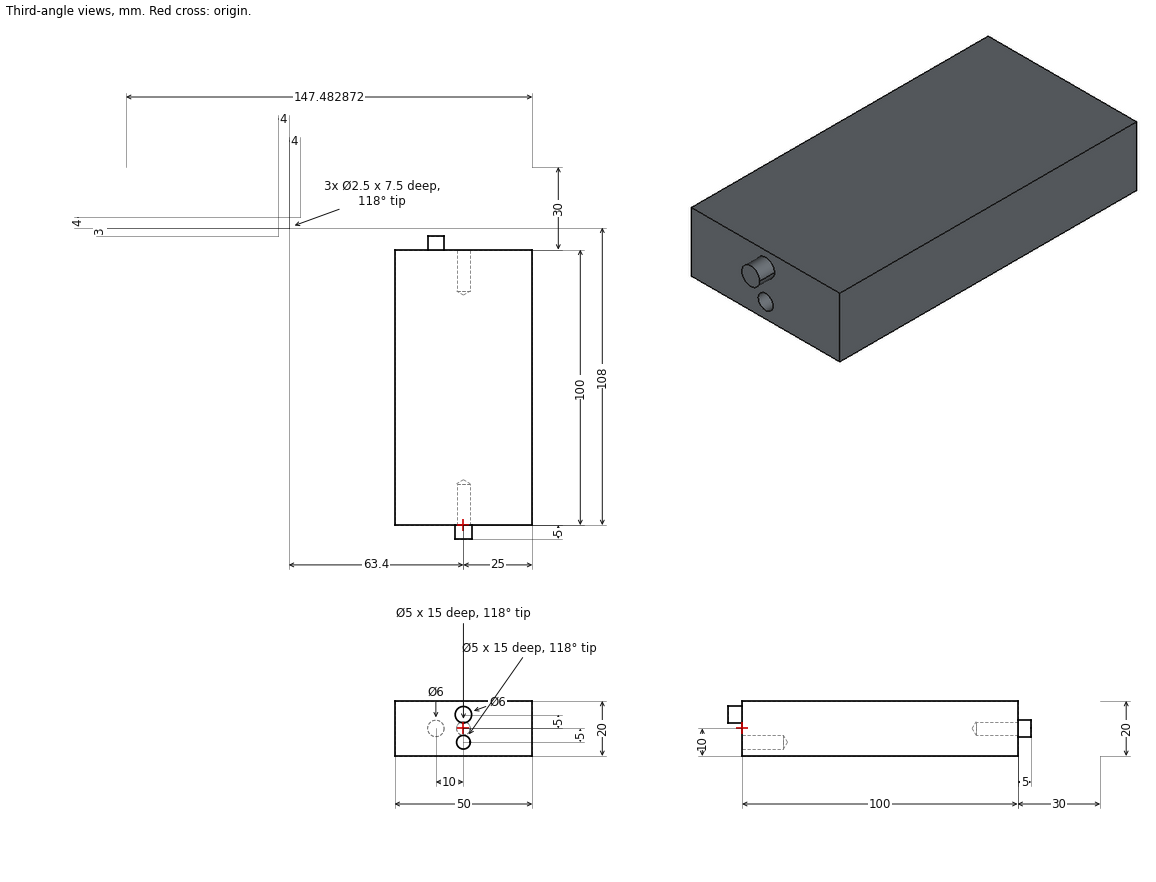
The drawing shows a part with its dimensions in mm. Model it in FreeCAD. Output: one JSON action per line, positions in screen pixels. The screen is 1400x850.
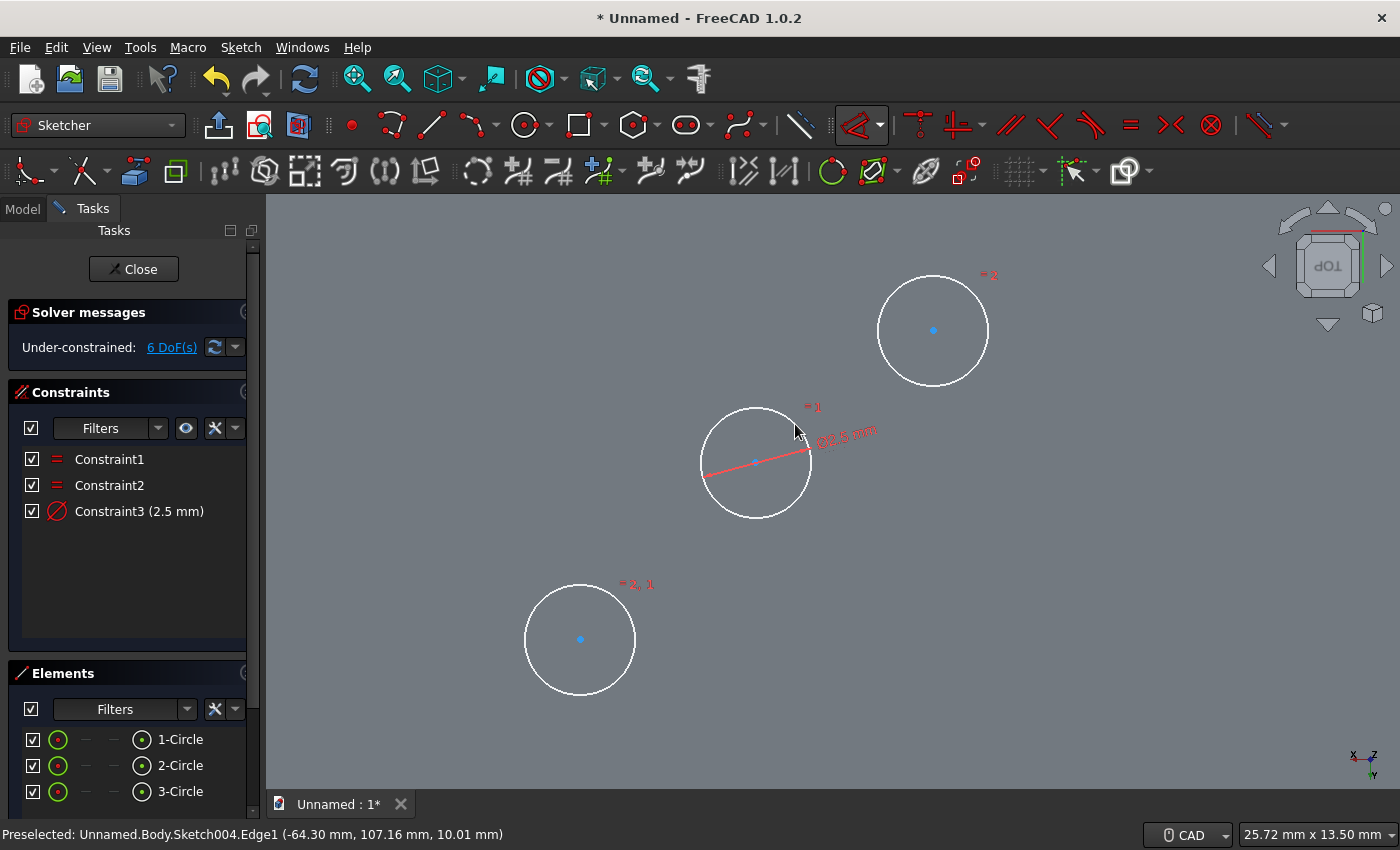
{"action": "left_click", "coordinate": [756, 463]}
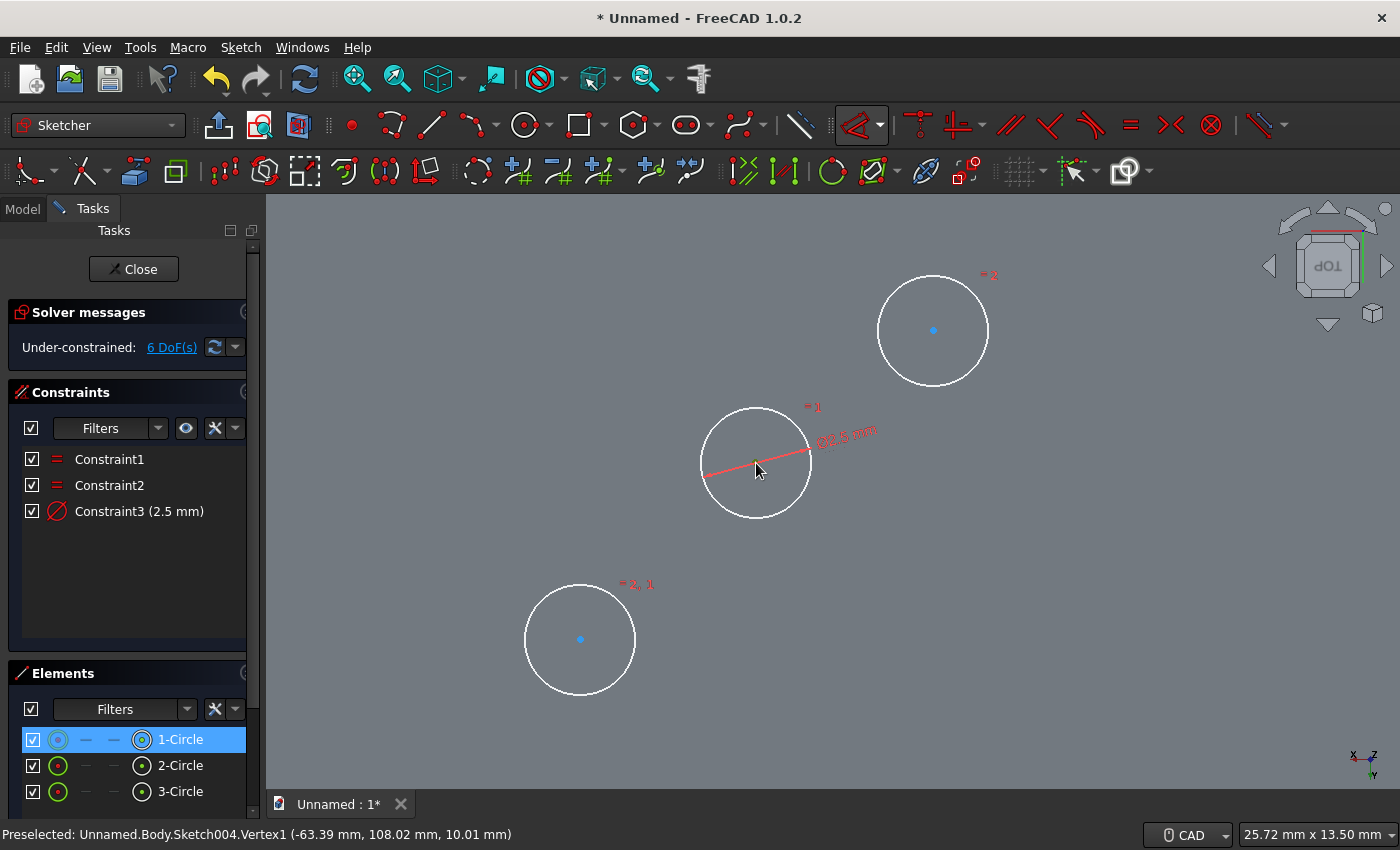
{"action": "left_click", "coordinate": [580, 640]}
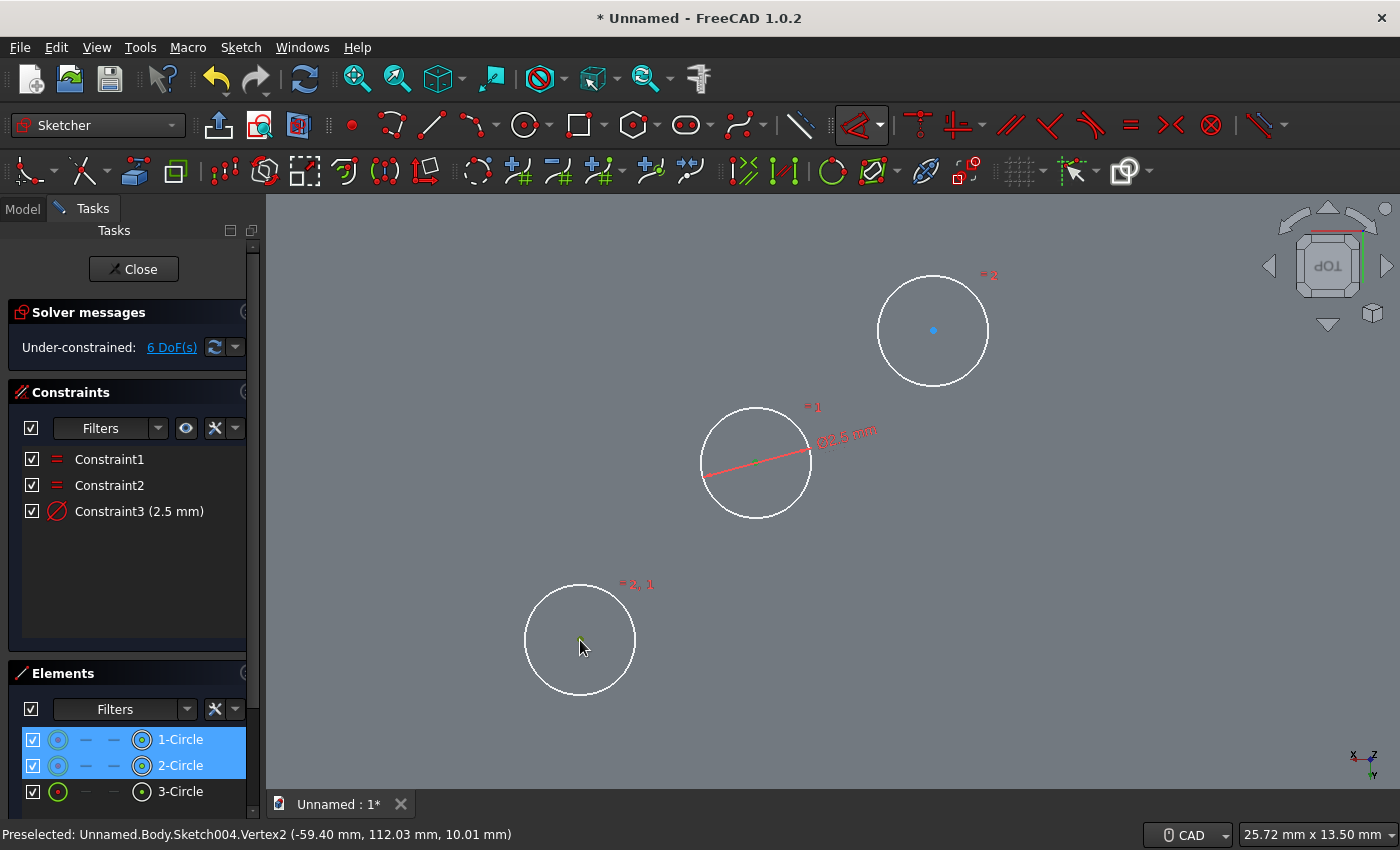
{"action": "left_click", "coordinate": [882, 126]}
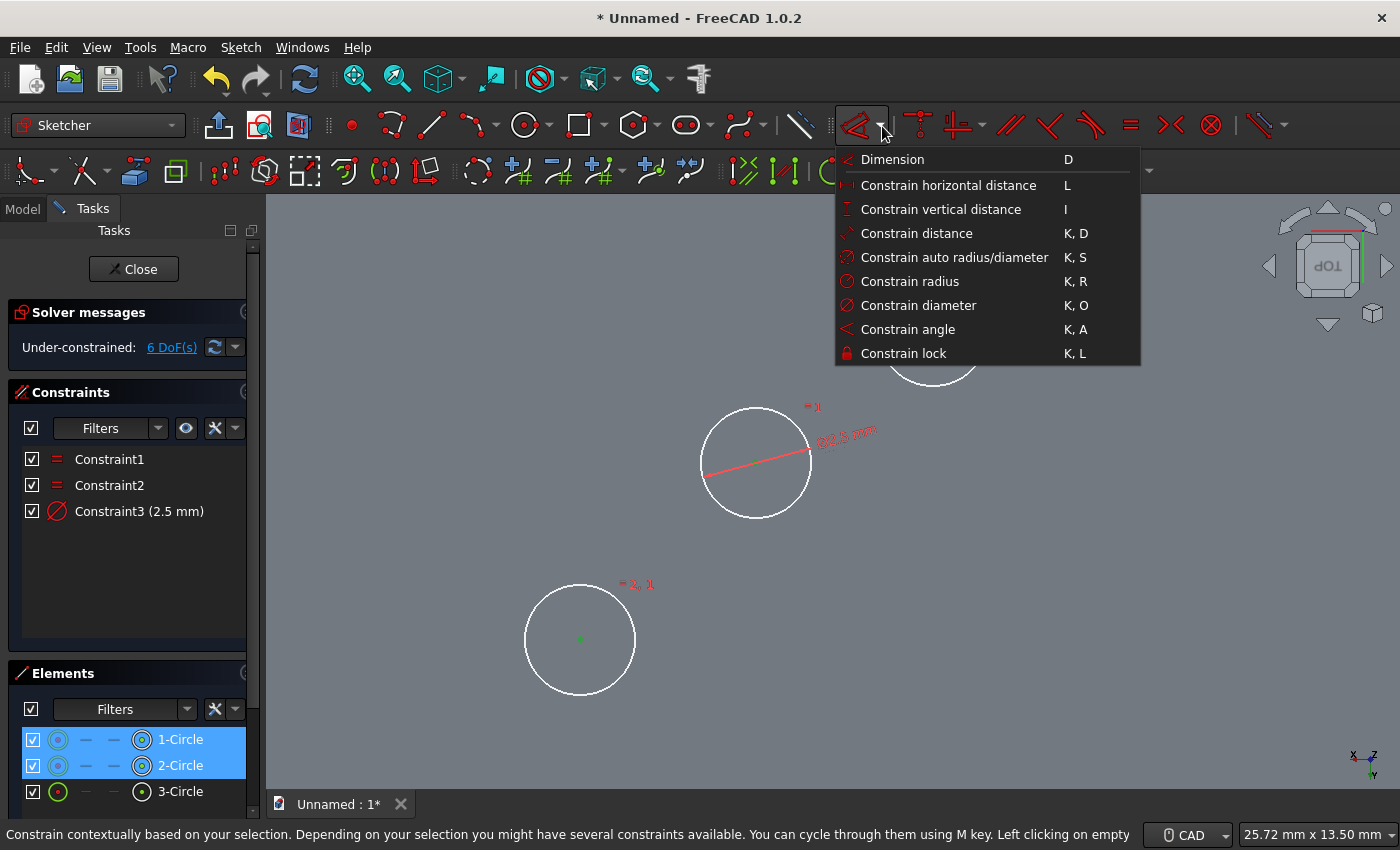
{"action": "left_click", "coordinate": [988, 185]}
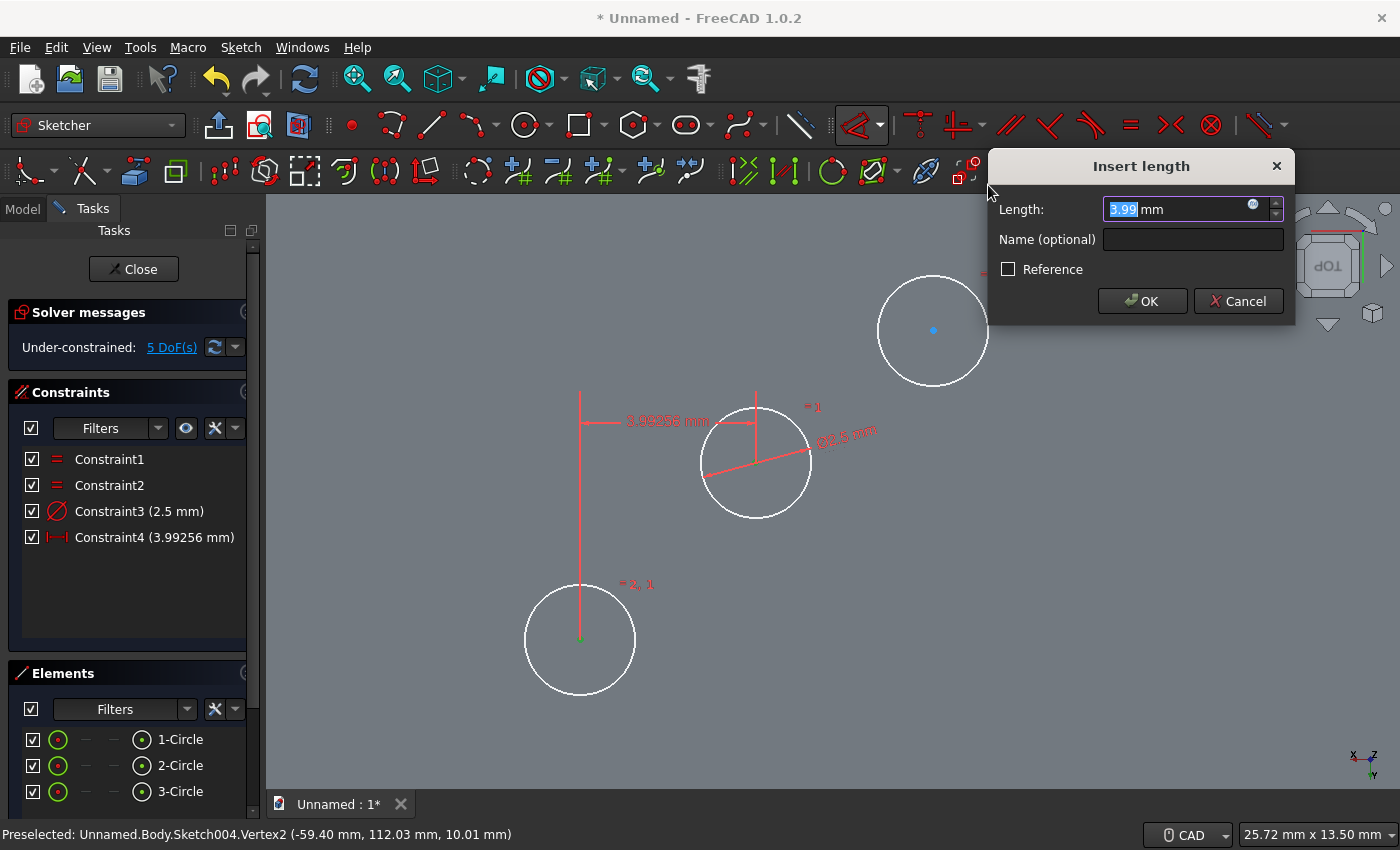
{"action": "type", "text": "4"}
{"action": "key", "text": "Return"}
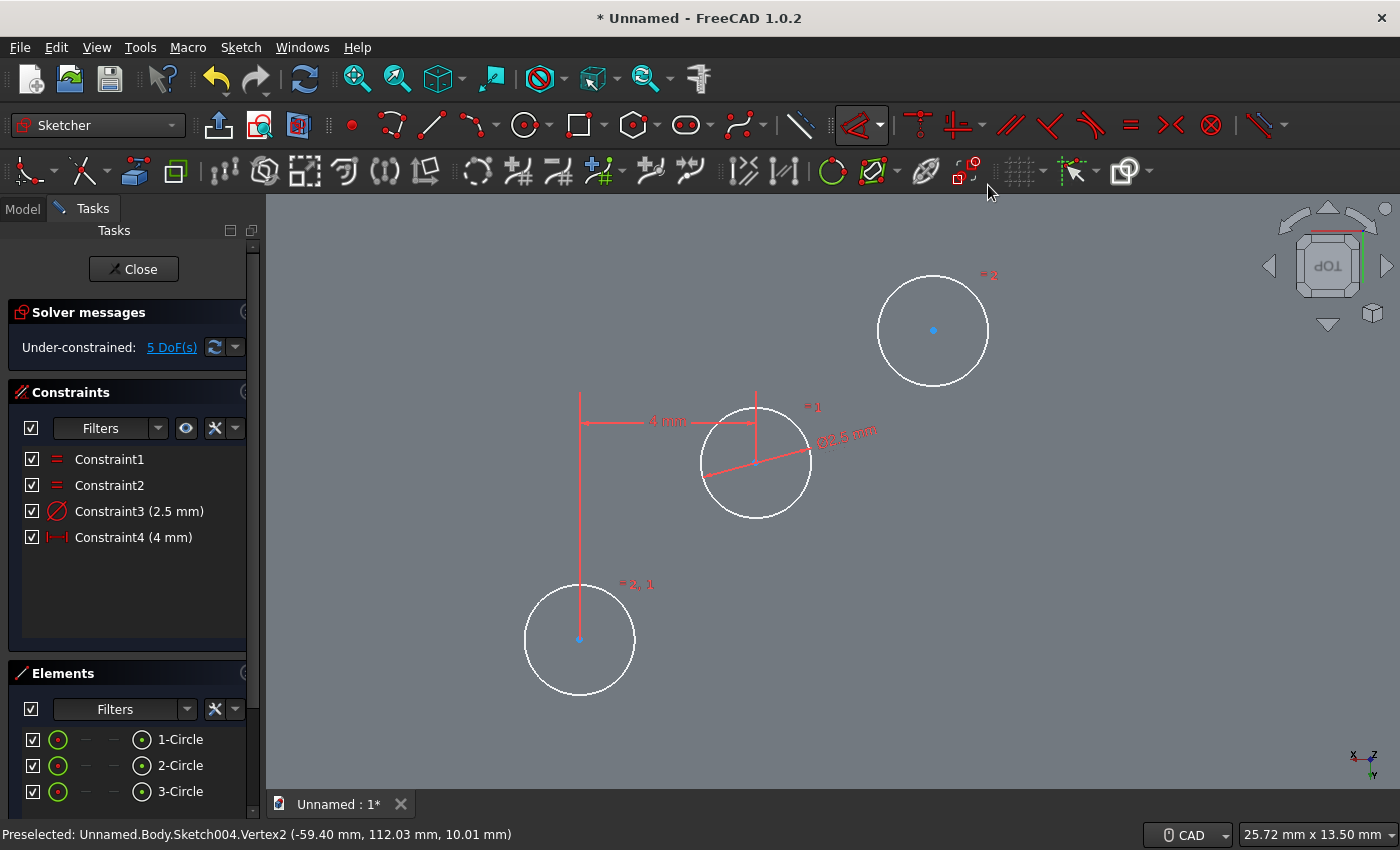
{"action": "left_click", "coordinate": [756, 463]}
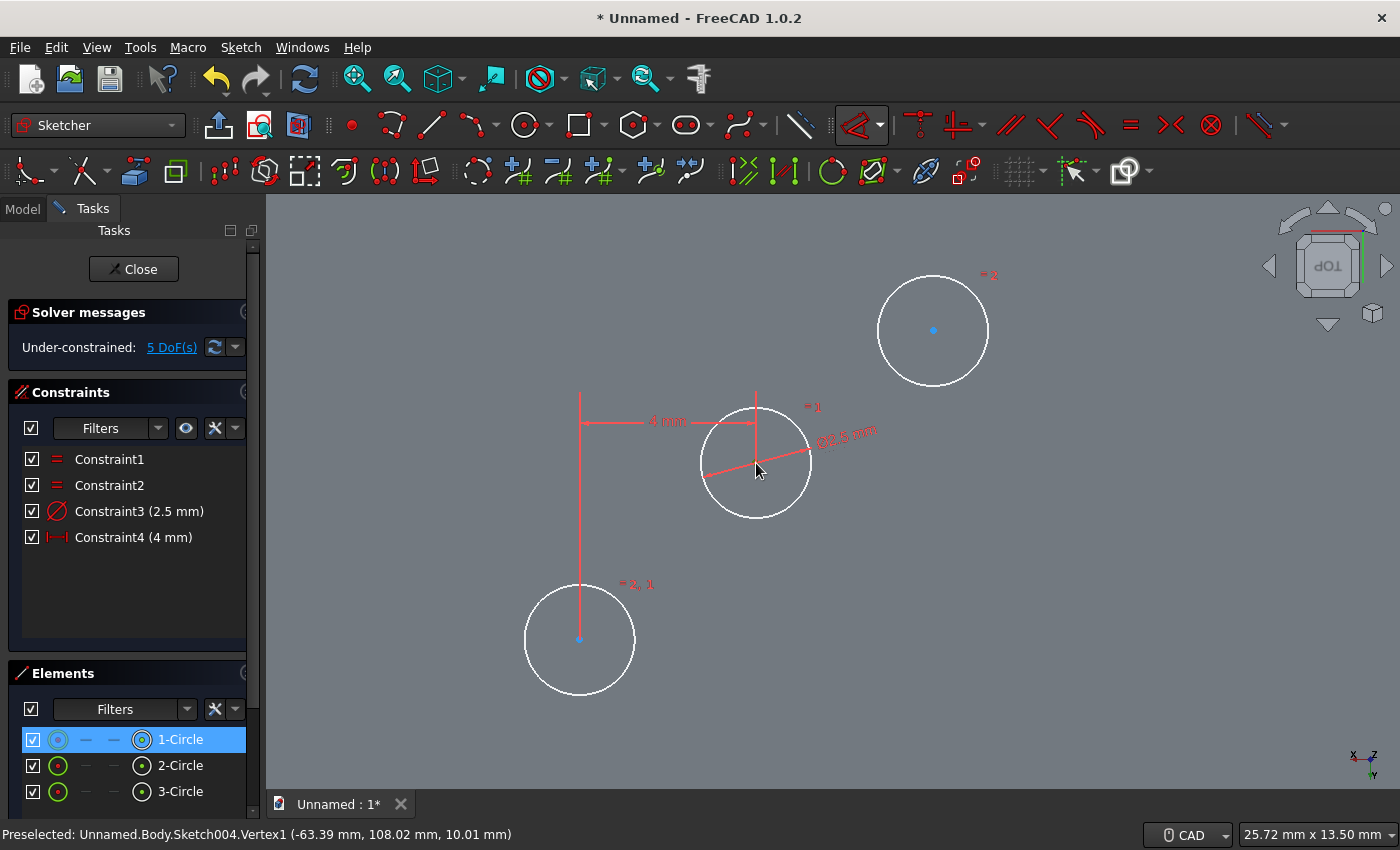
{"action": "left_click", "coordinate": [580, 640]}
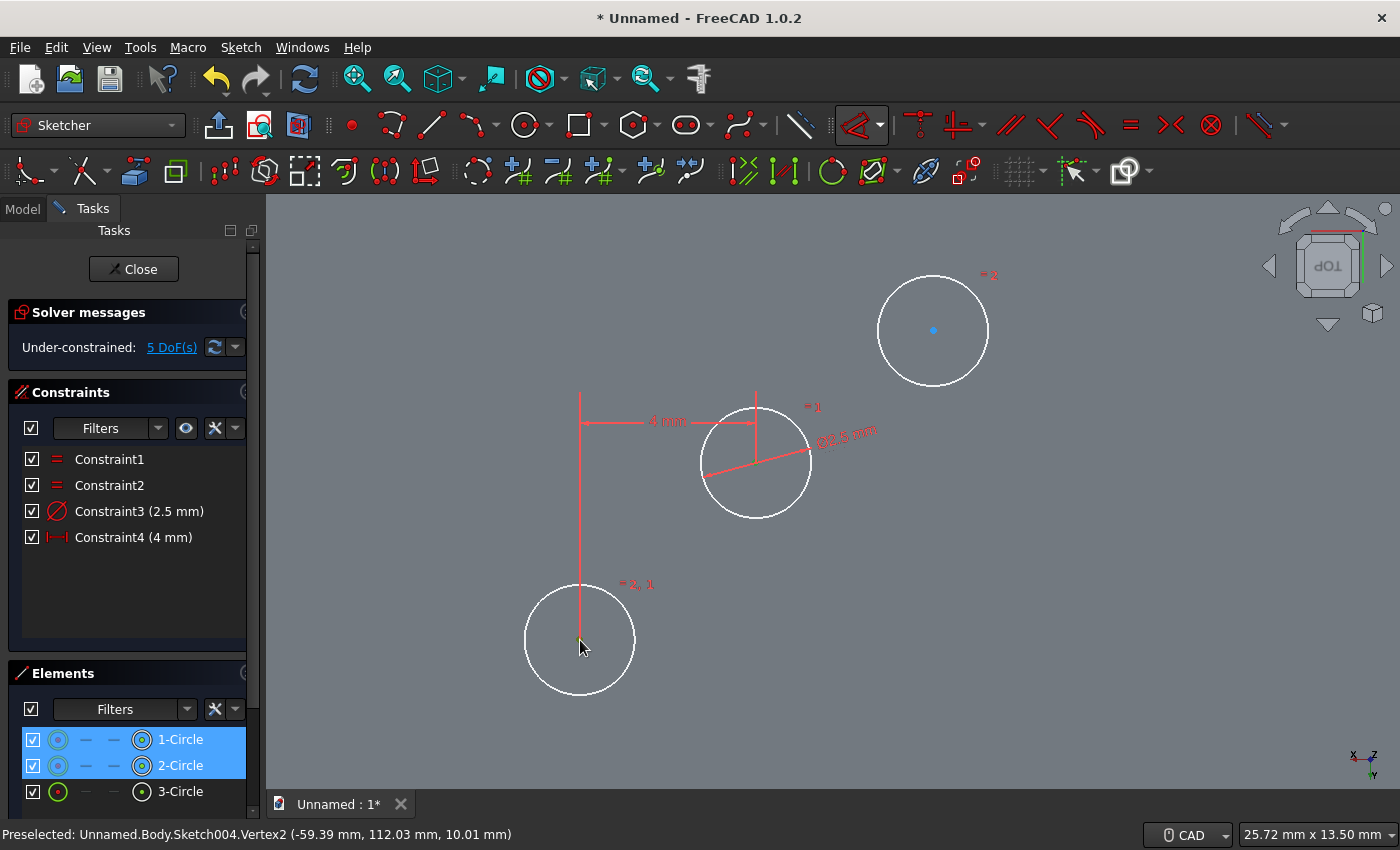
{"action": "key", "text": "i"}